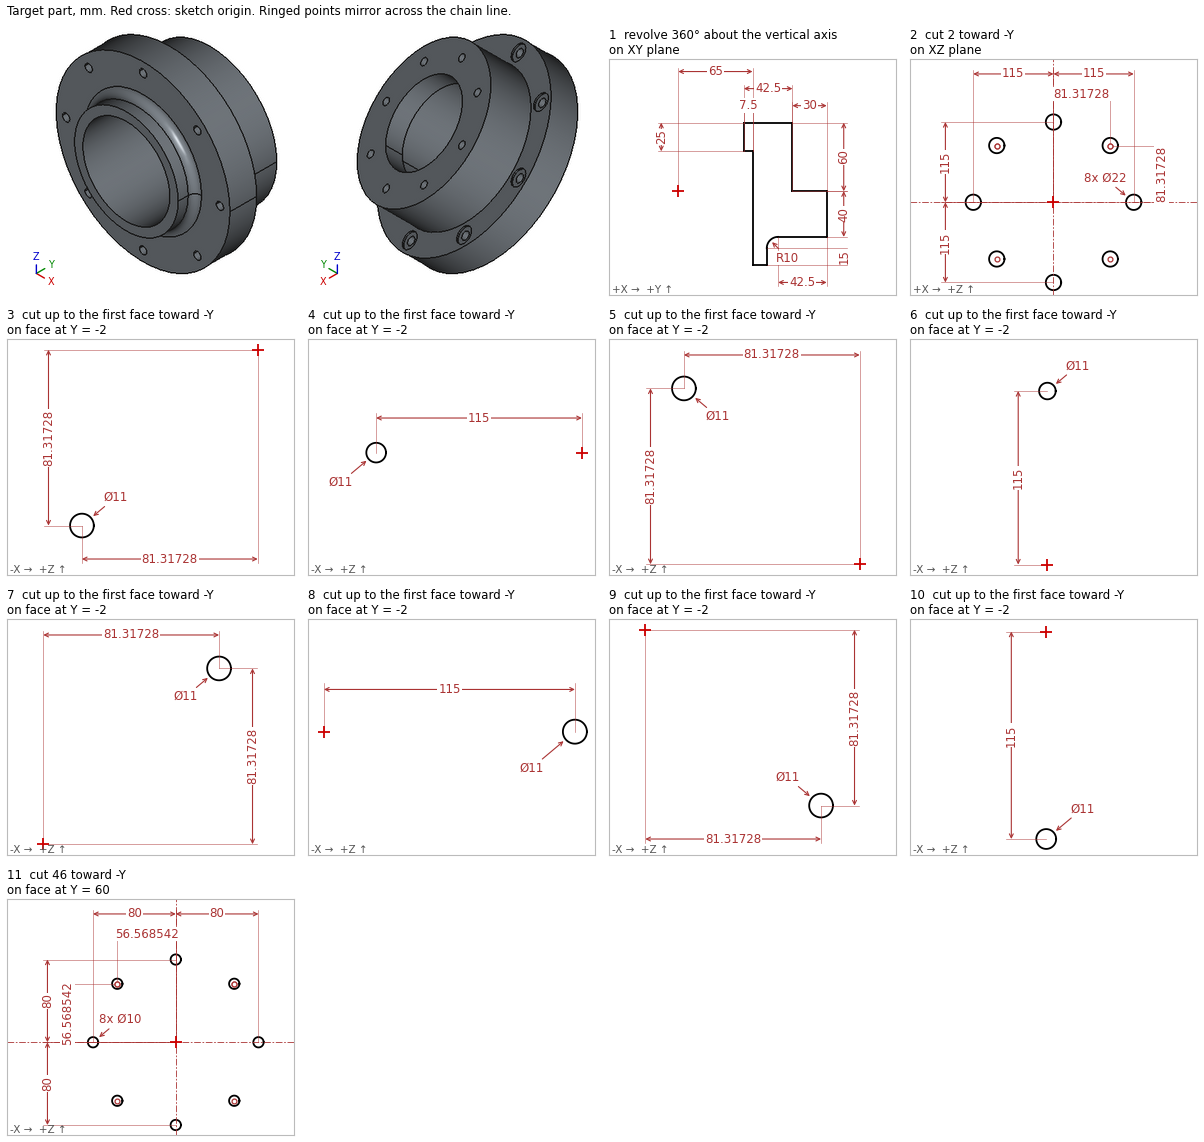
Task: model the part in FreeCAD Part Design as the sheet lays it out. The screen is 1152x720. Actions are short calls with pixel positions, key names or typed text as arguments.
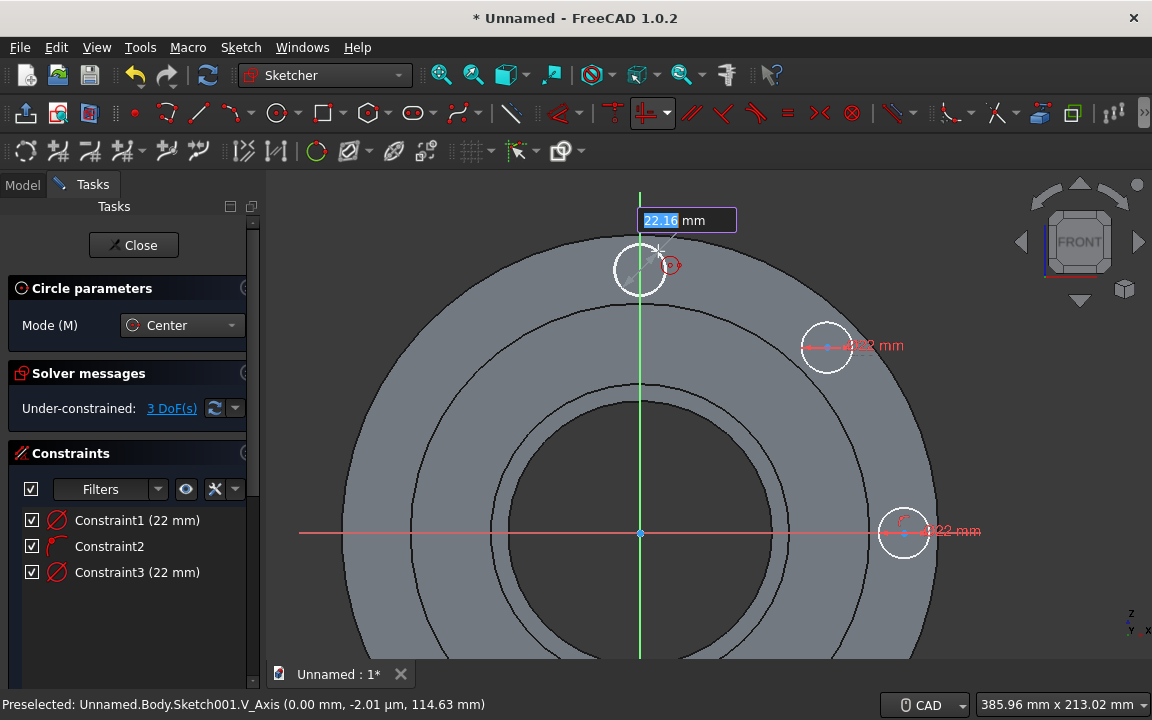
text(22)
key(Return)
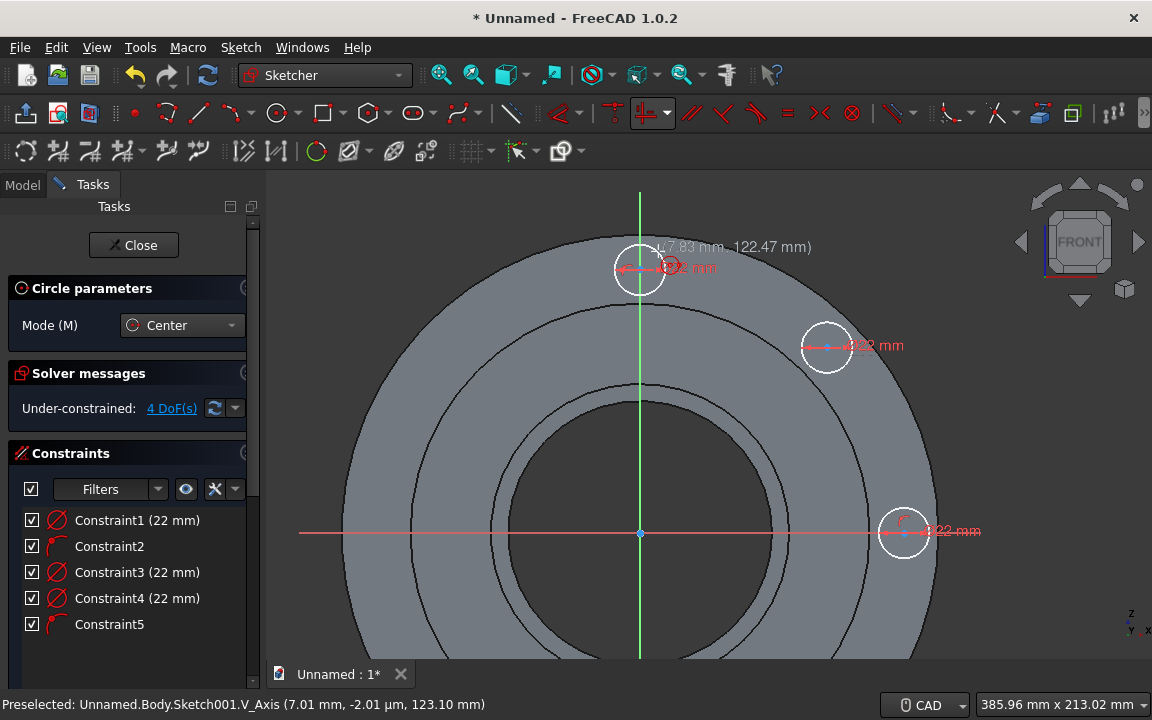
click(453, 346)
move(471, 329)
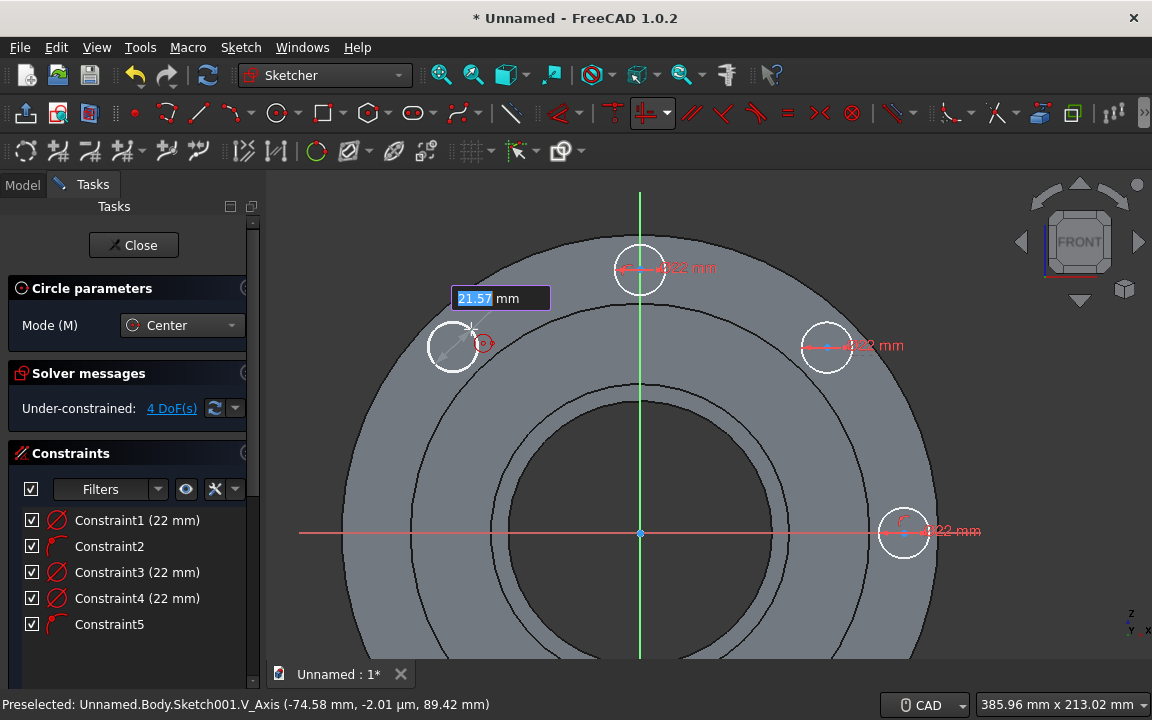
text(22)
key(Return)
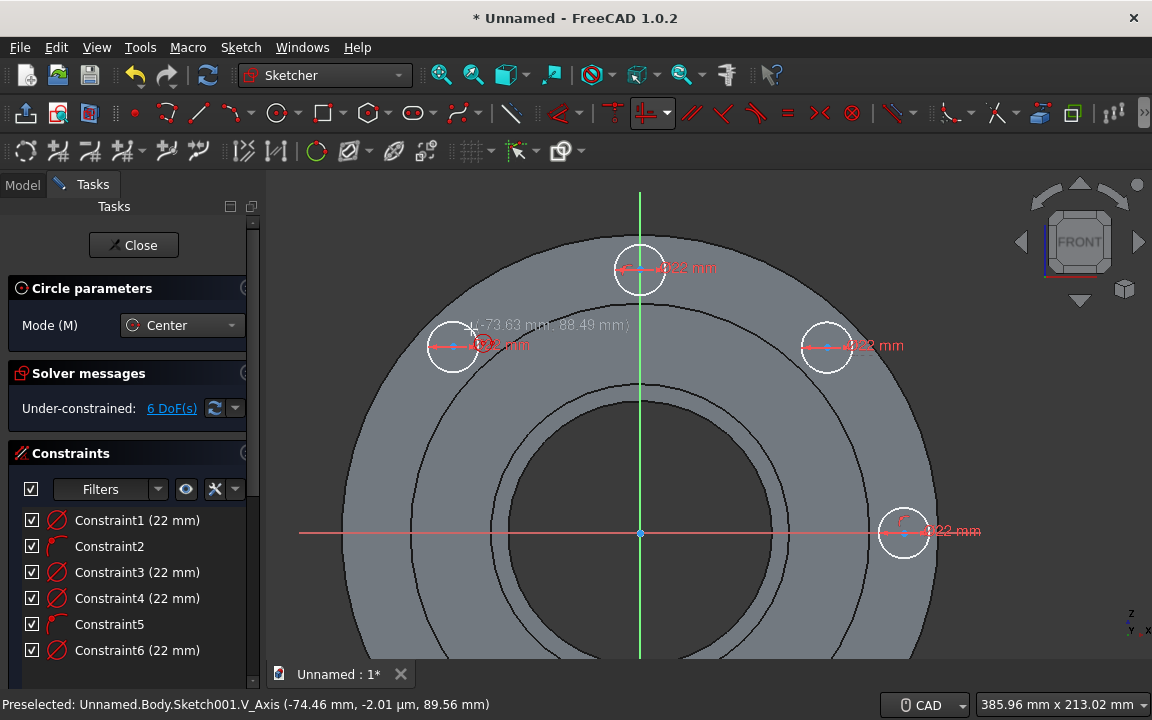
click(376, 533)
move(394, 515)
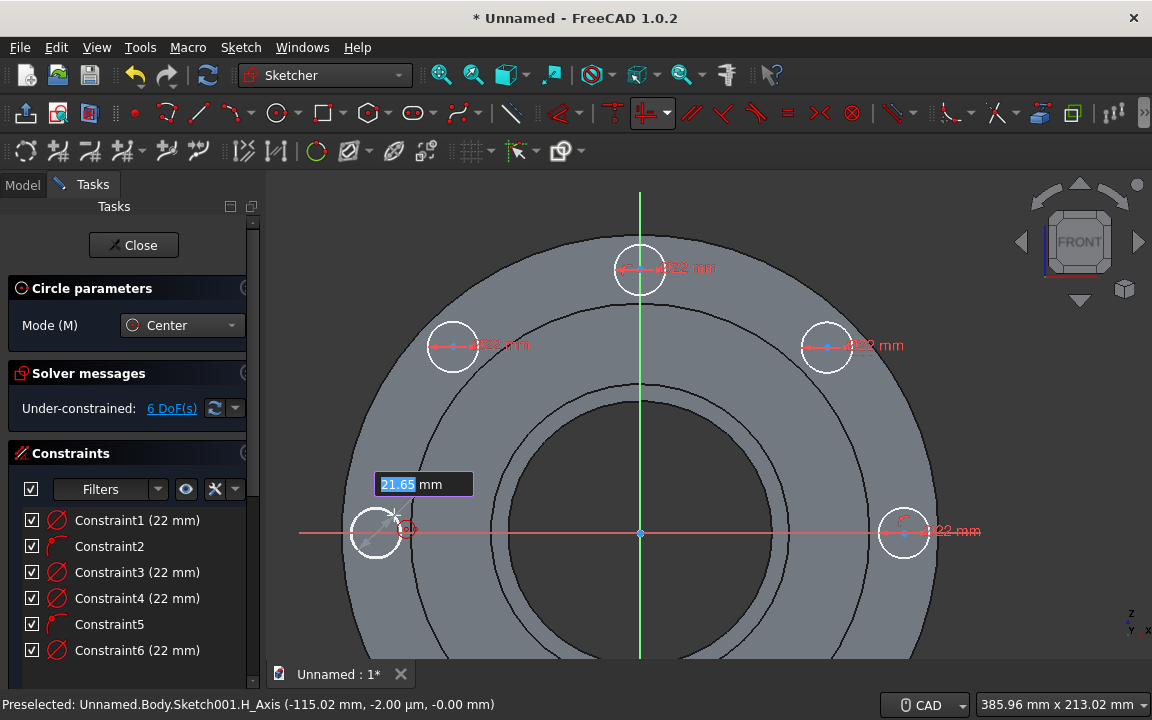
text(22)
key(Return)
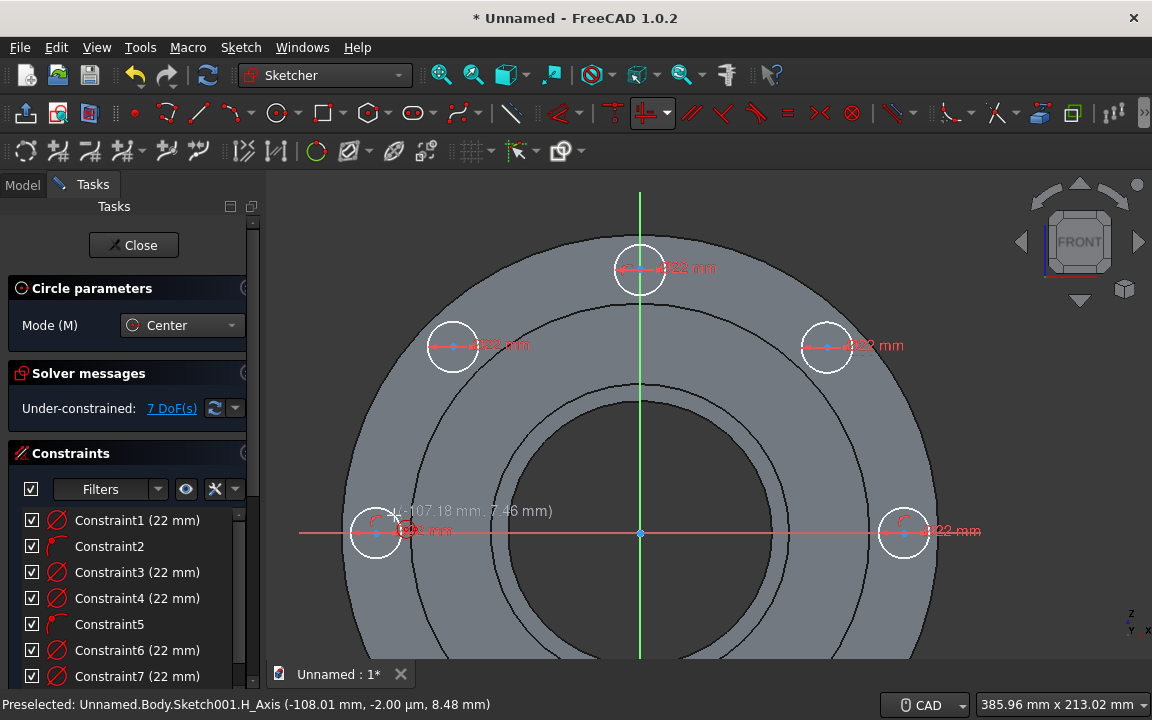
scroll(641, 270, down, 3)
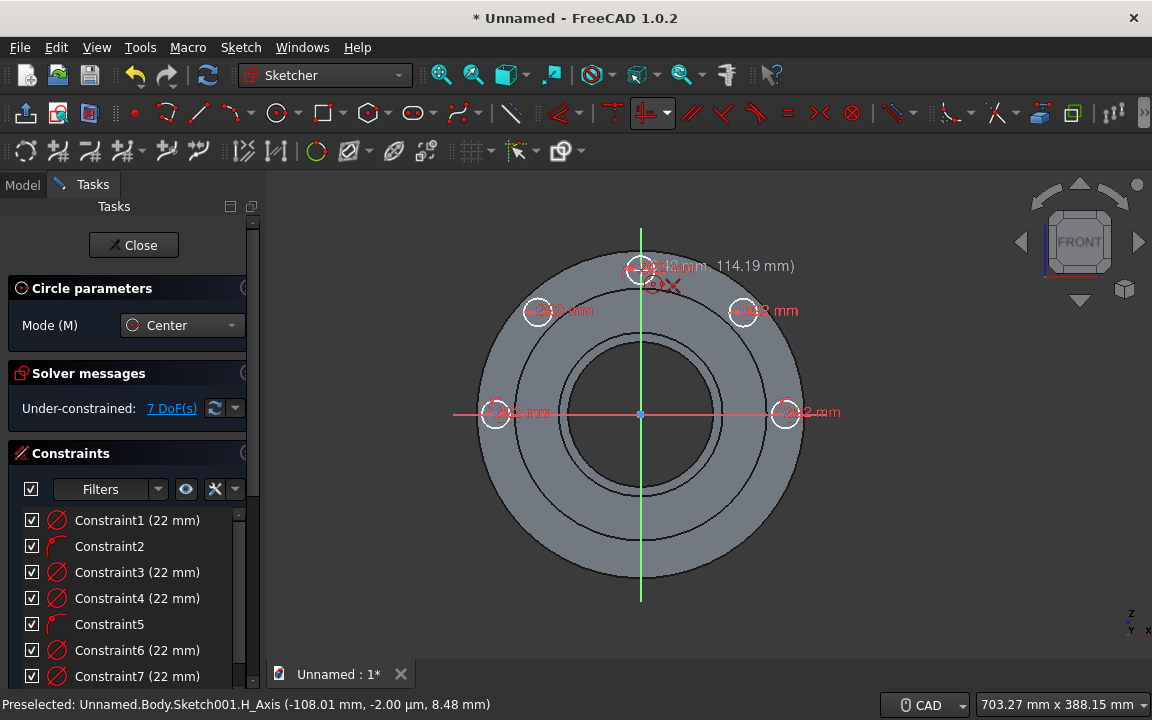
scroll(538, 517, up, 3)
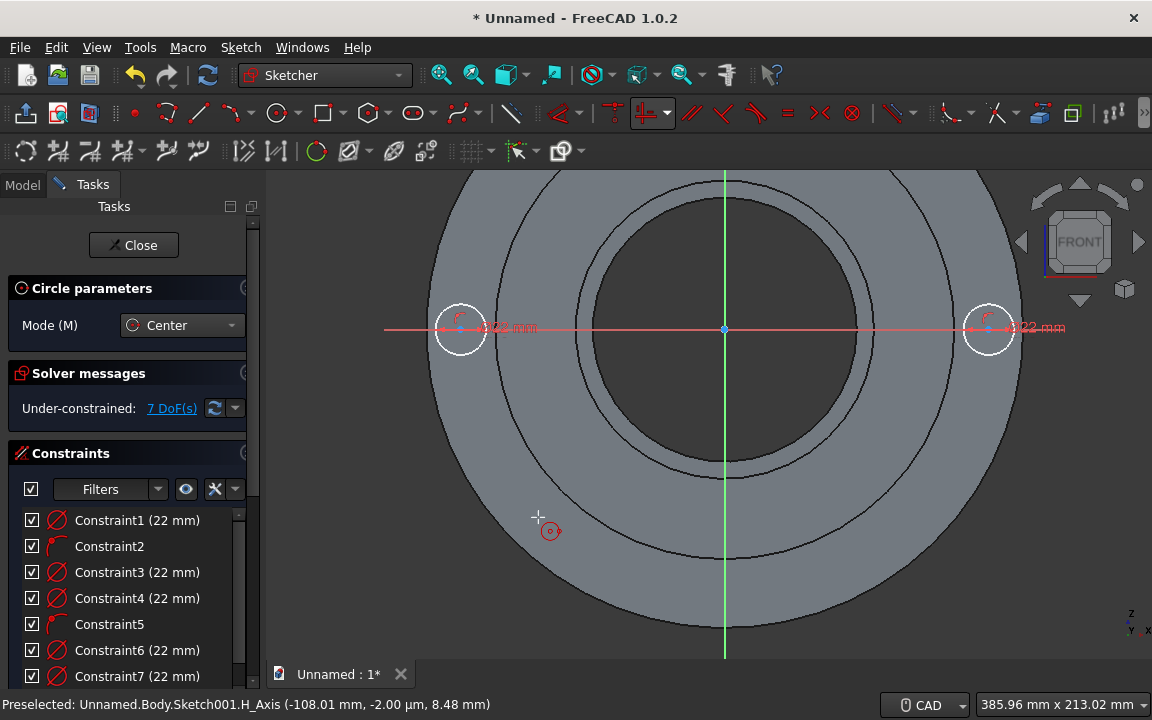
click(538, 516)
move(556, 498)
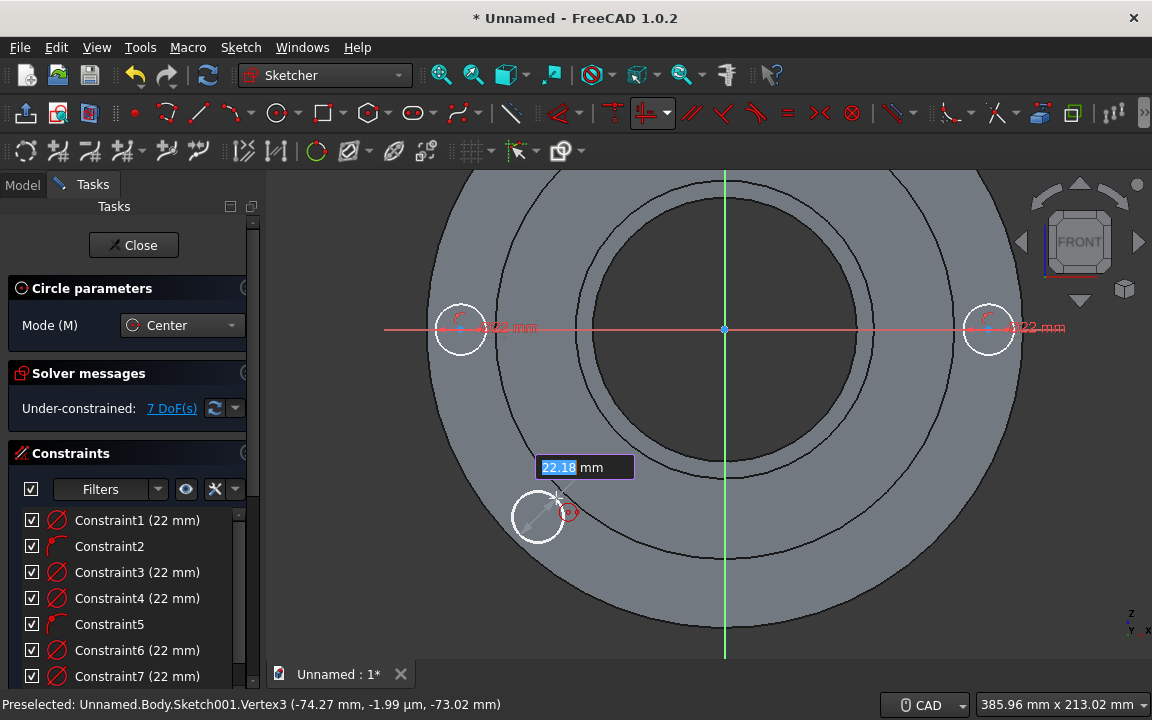
text(22)
key(Return)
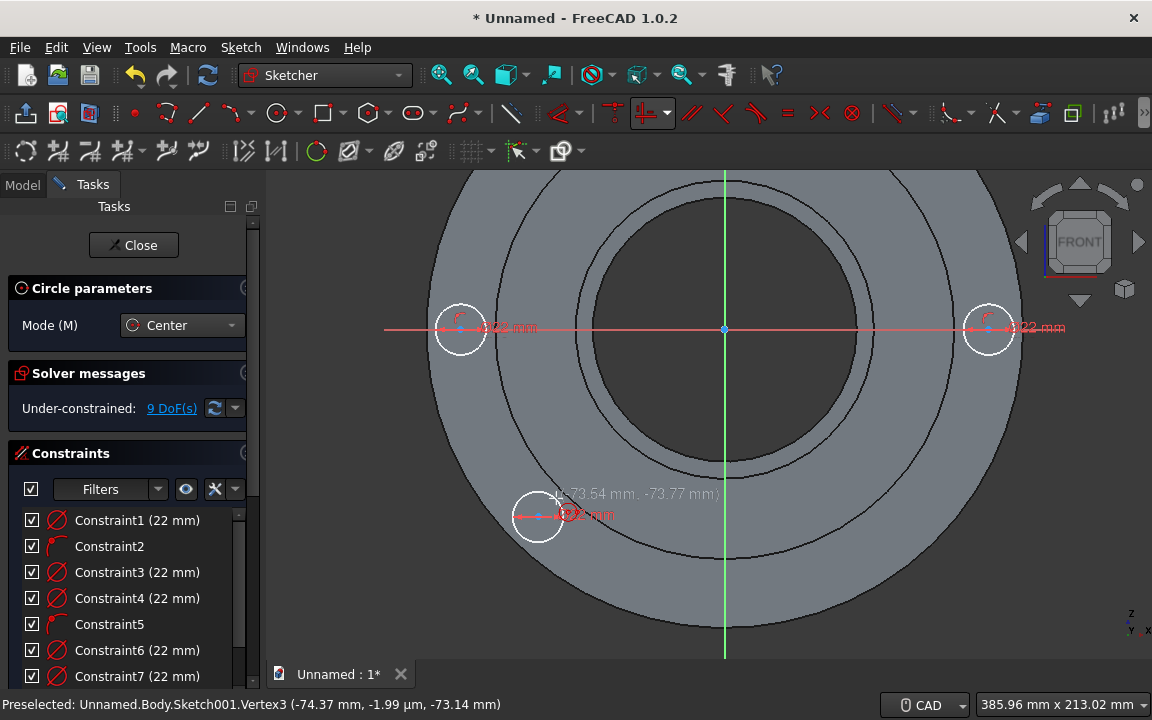
click(725, 594)
move(743, 576)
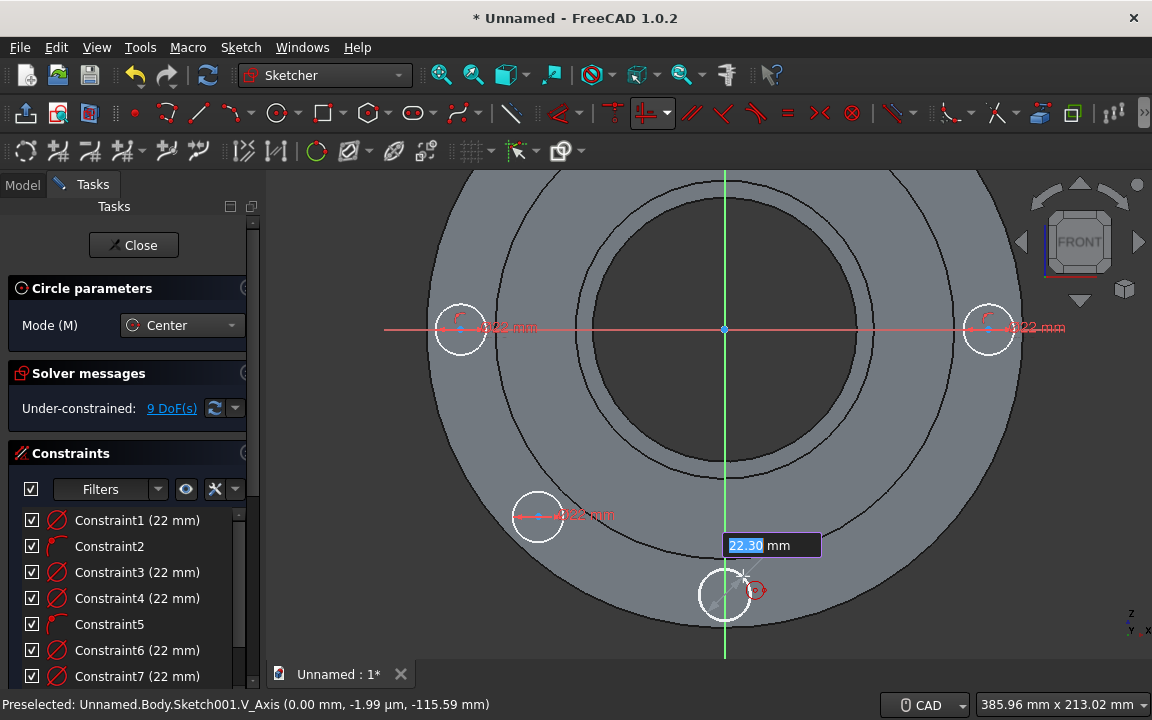
text(22)
key(Return)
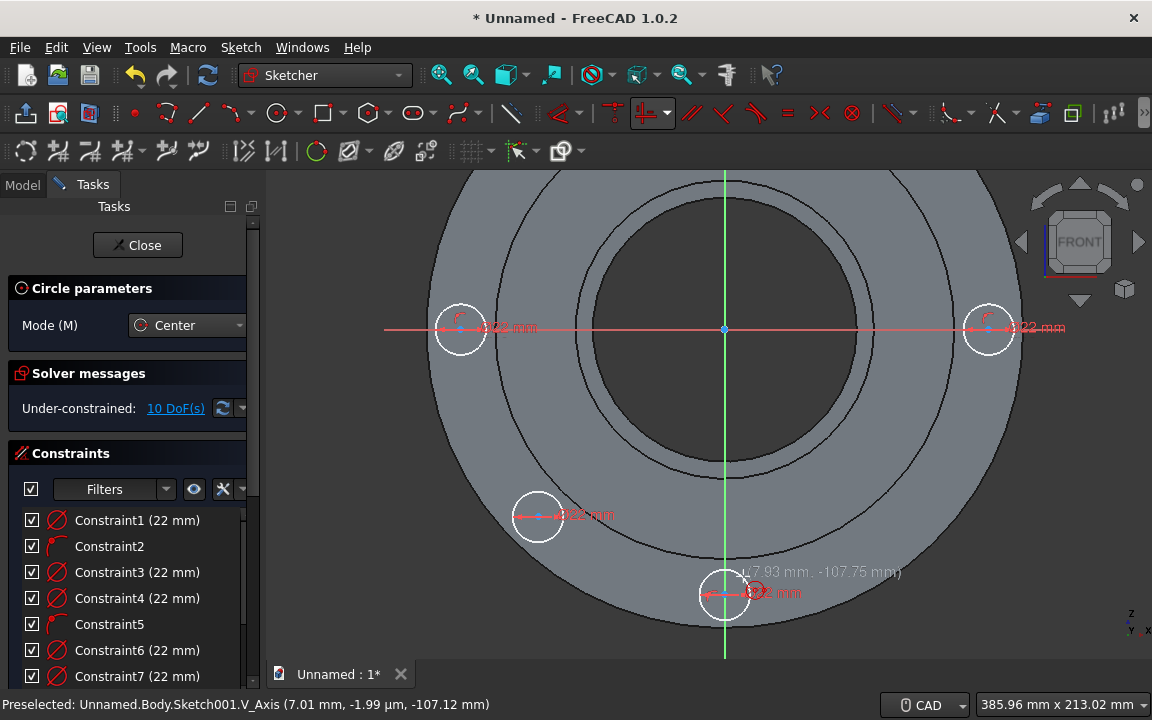
click(911, 516)
move(929, 498)